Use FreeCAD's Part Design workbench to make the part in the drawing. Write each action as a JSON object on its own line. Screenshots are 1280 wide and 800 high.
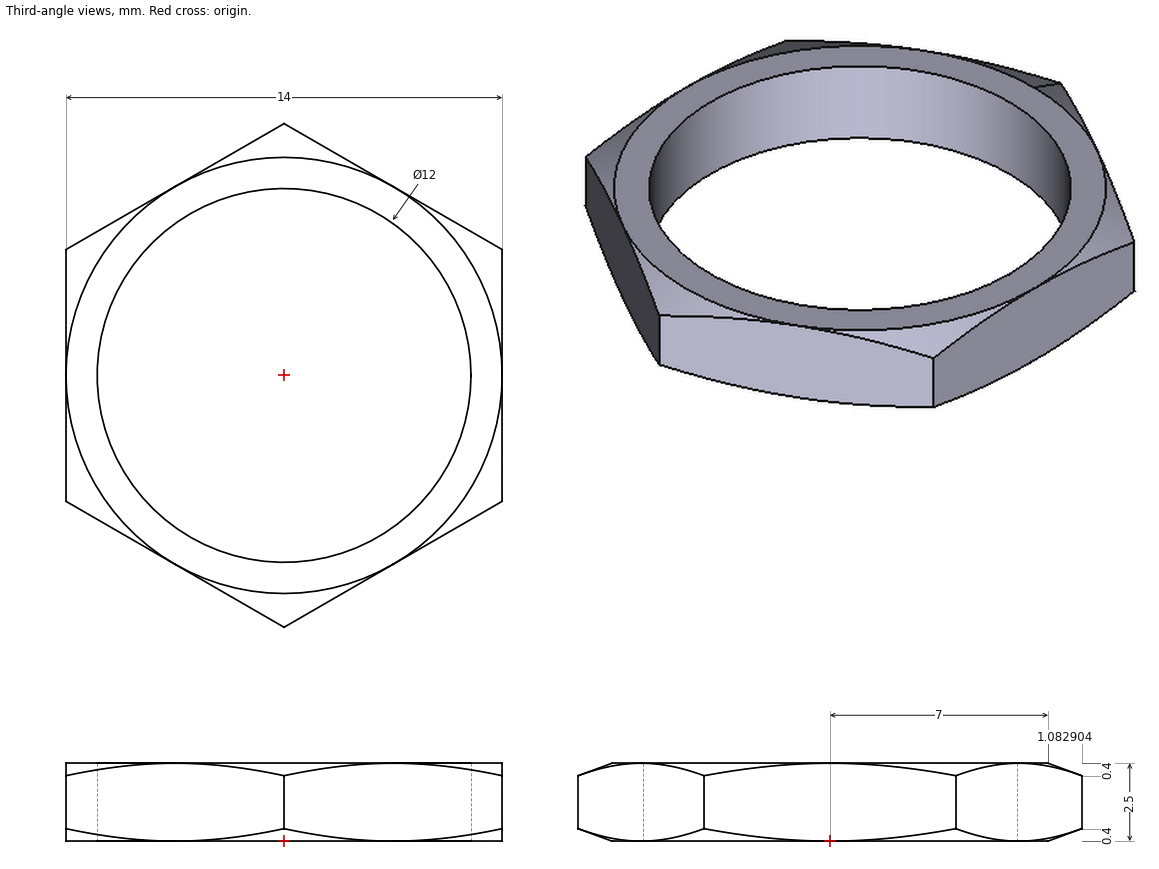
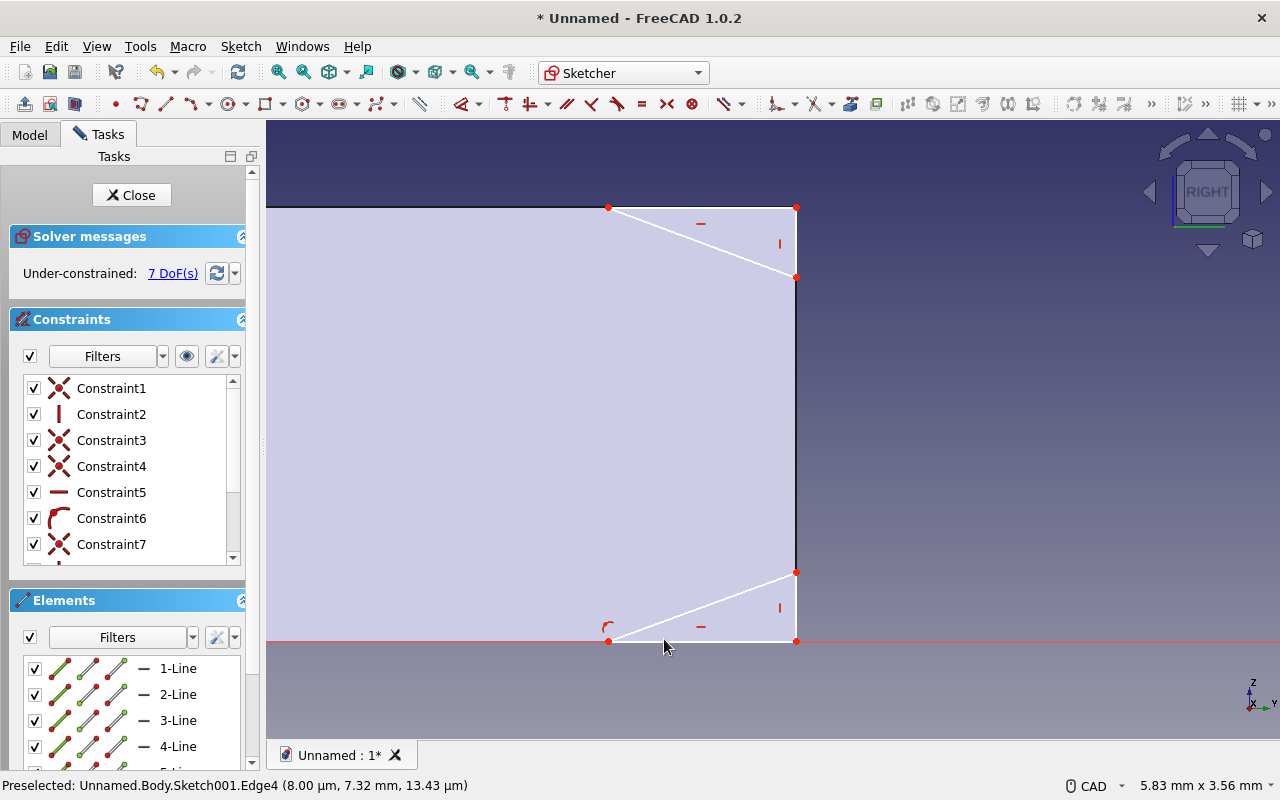
{"action": "key", "text": "d"}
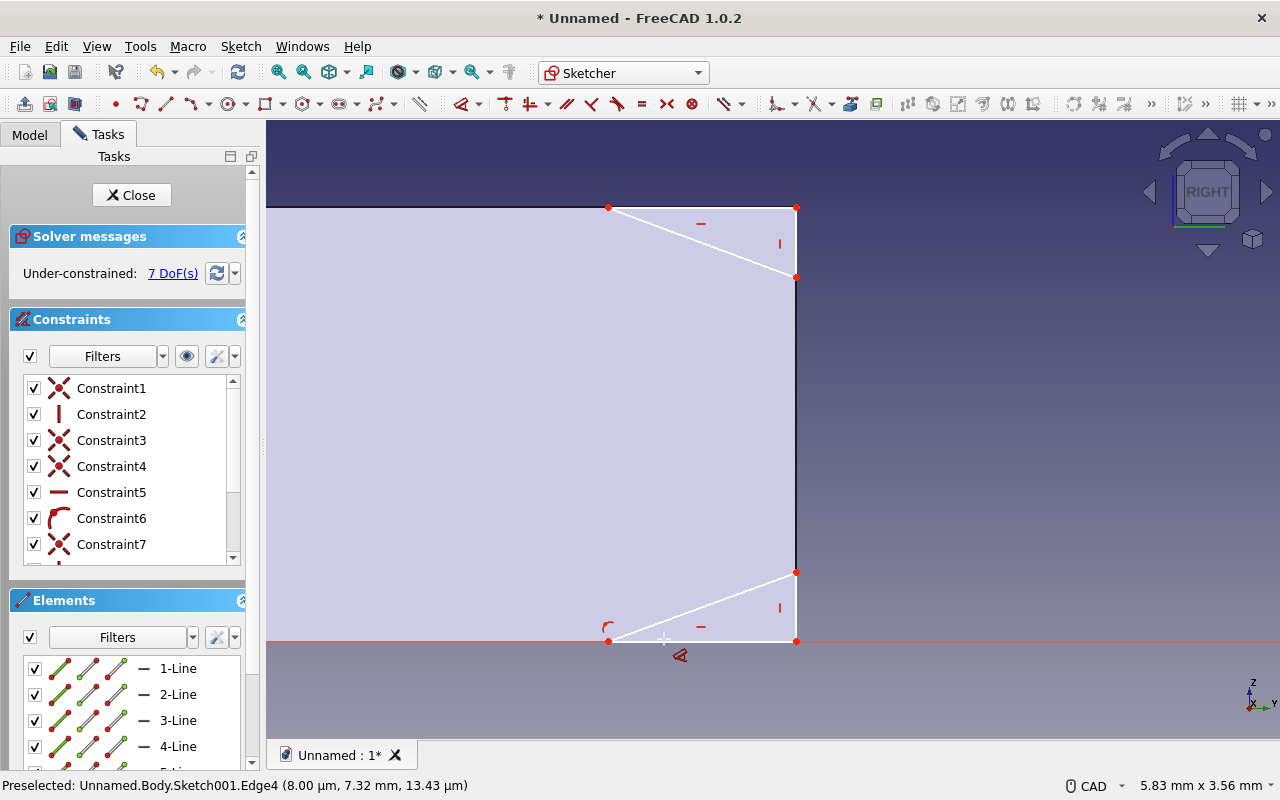
{"action": "left_click", "coordinate": [608, 208]}
{"action": "left_click", "coordinate": [451, 676]}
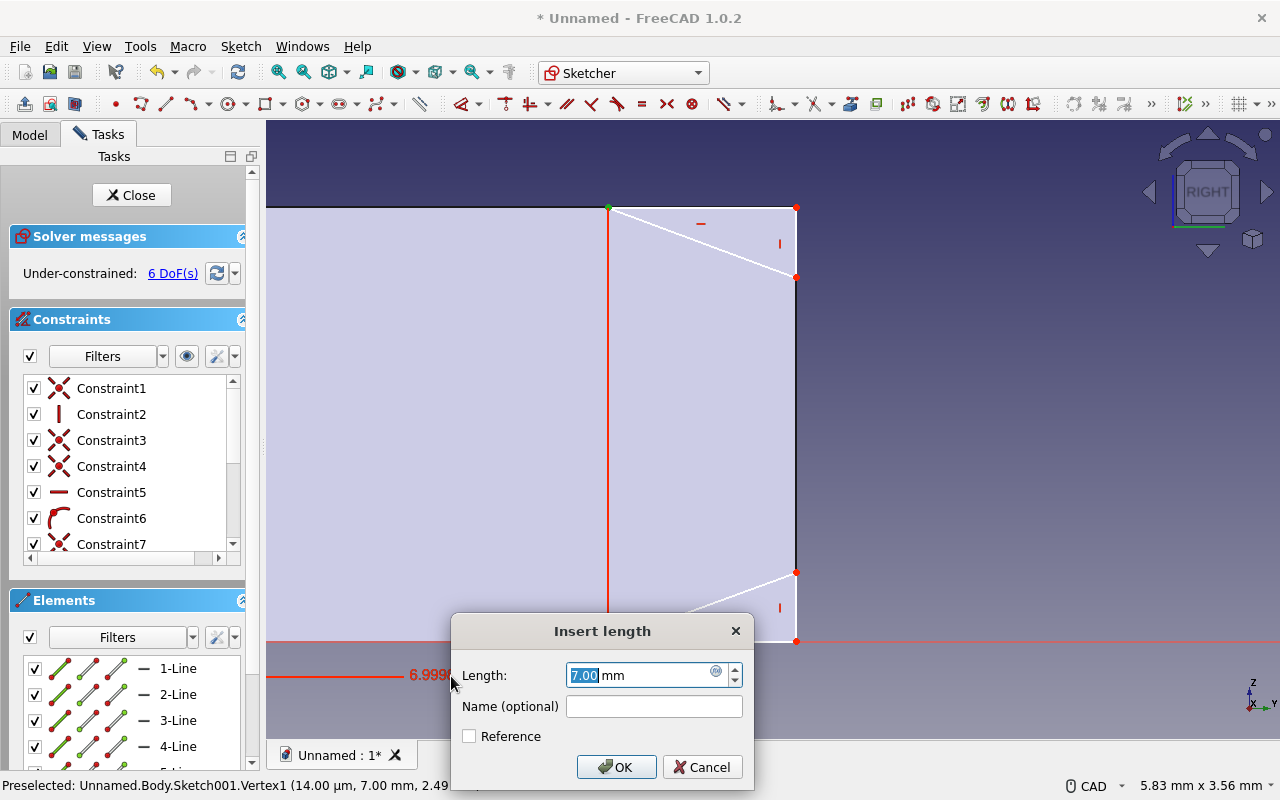
{"action": "type", "text": "7"}
{"action": "key", "text": "Return"}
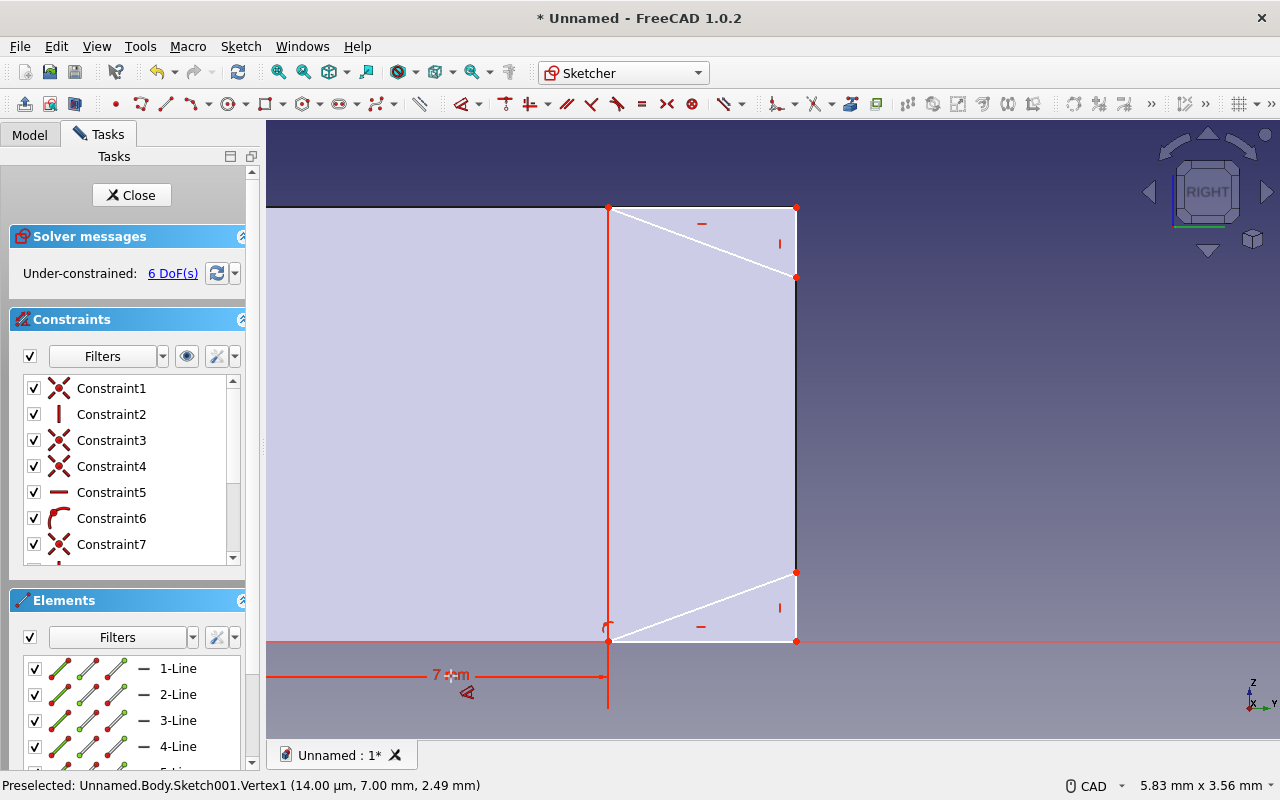
{"action": "left_click", "coordinate": [608, 642]}
{"action": "left_click", "coordinate": [379, 676]}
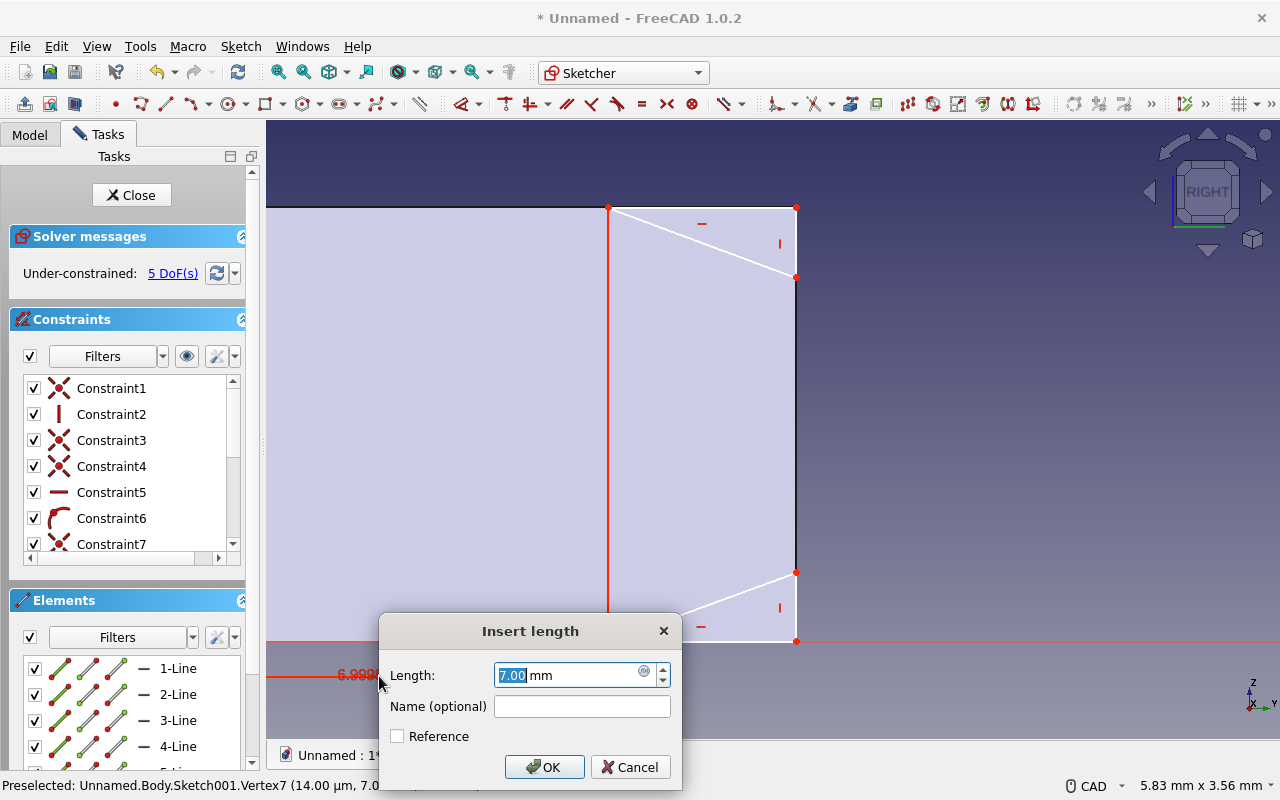
{"action": "type", "text": "7"}
{"action": "key", "text": "Return"}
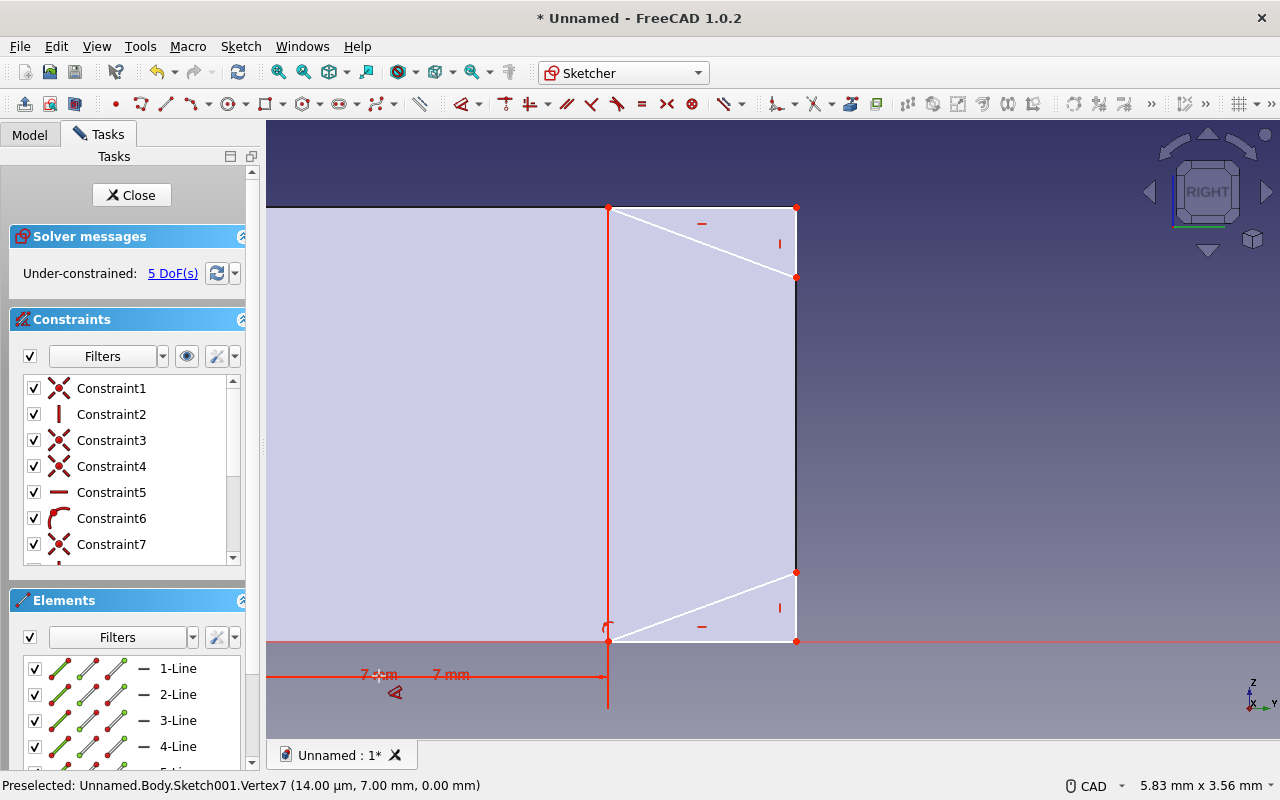
{"action": "left_click", "coordinate": [796, 257]}
{"action": "left_click", "coordinate": [830, 243]}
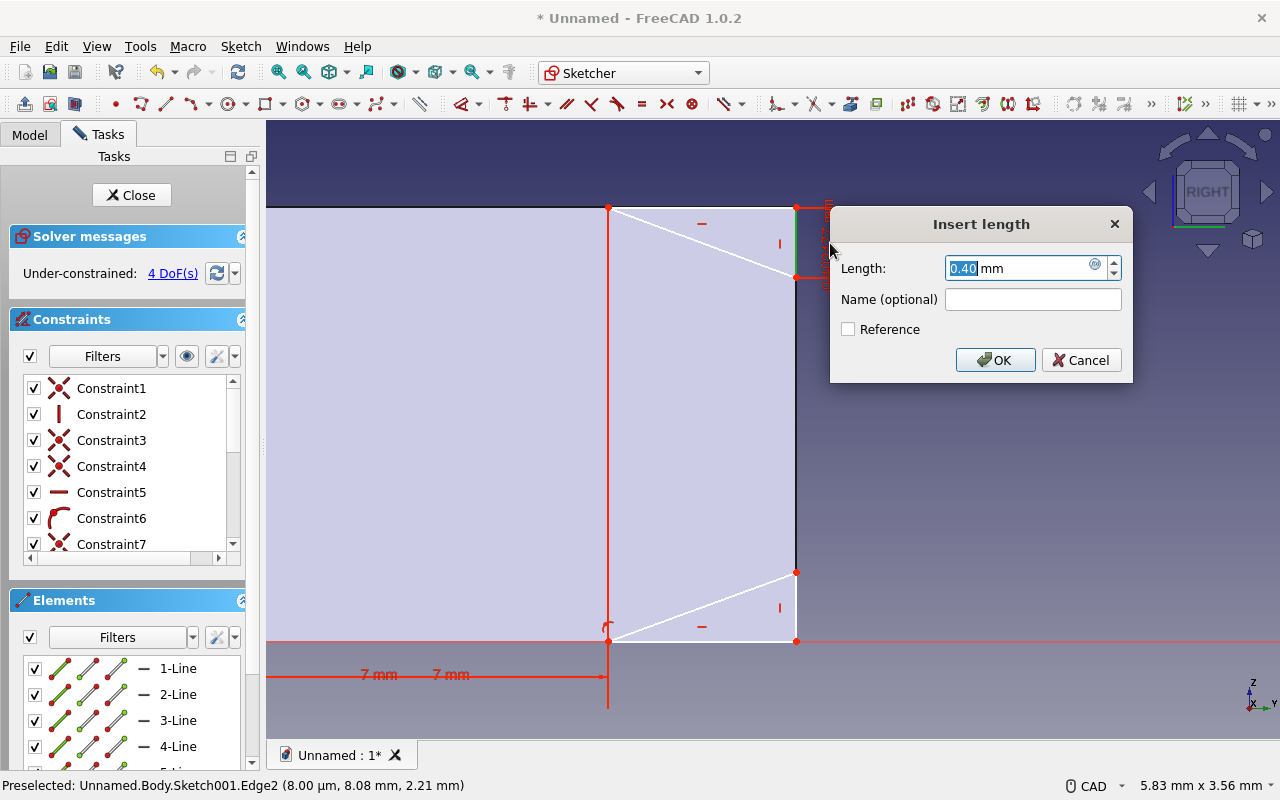
{"action": "type", "text": "0.4"}
{"action": "key", "text": "Return"}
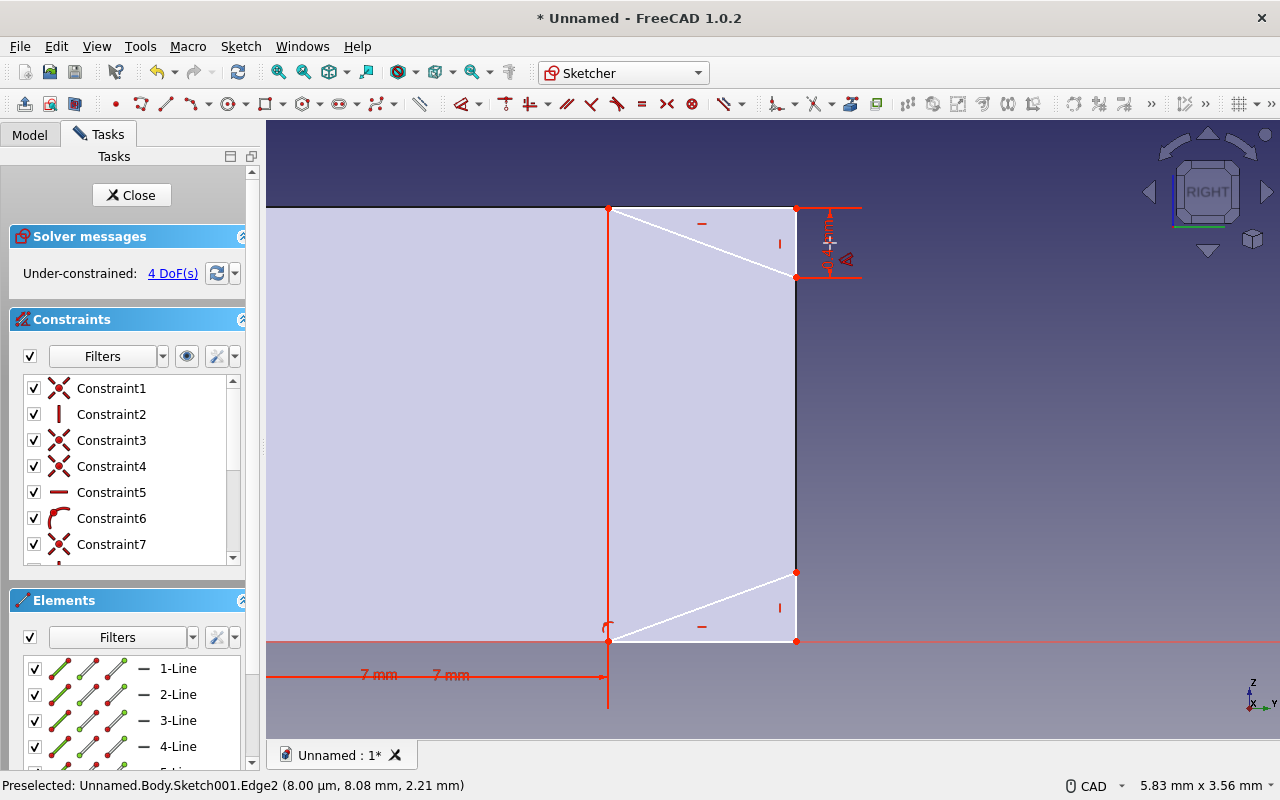
{"action": "left_click", "coordinate": [796, 621]}
{"action": "left_click", "coordinate": [830, 607]}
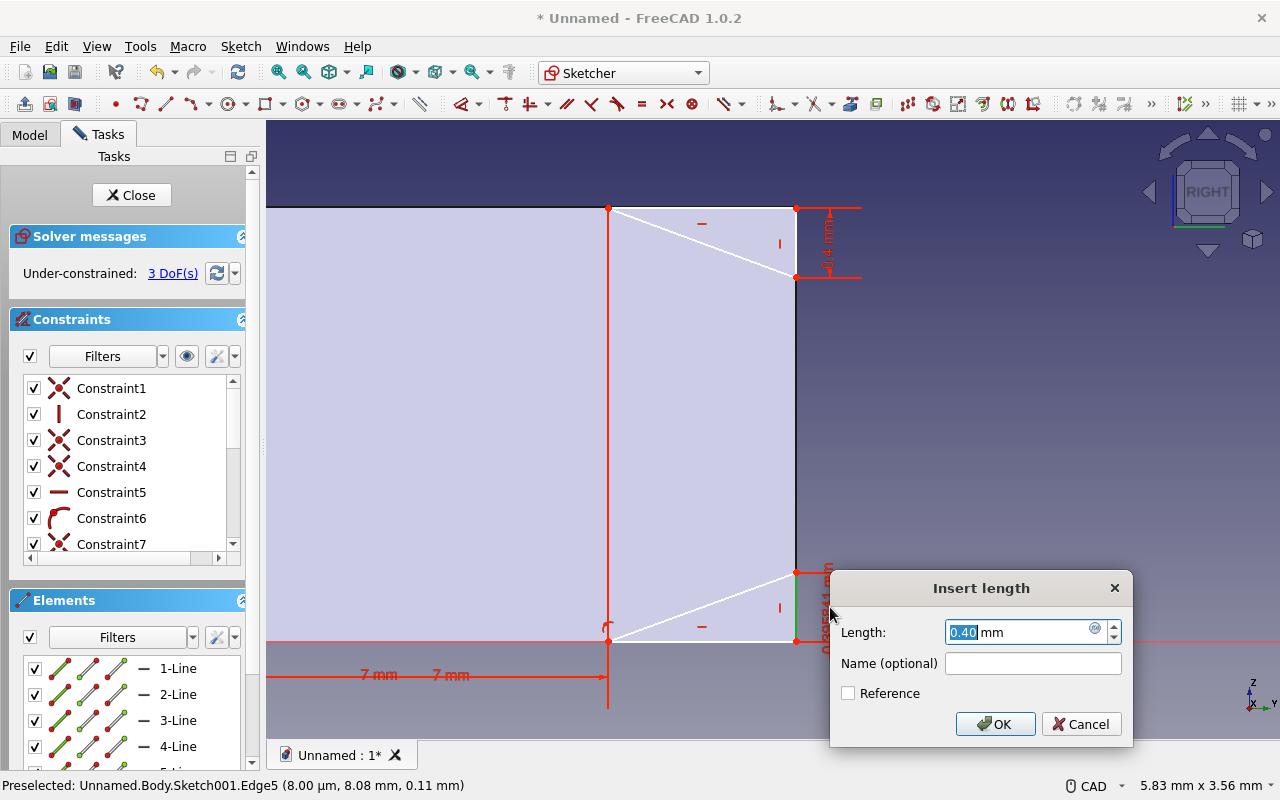
{"action": "type", "text": "0.4"}
{"action": "key", "text": "Return"}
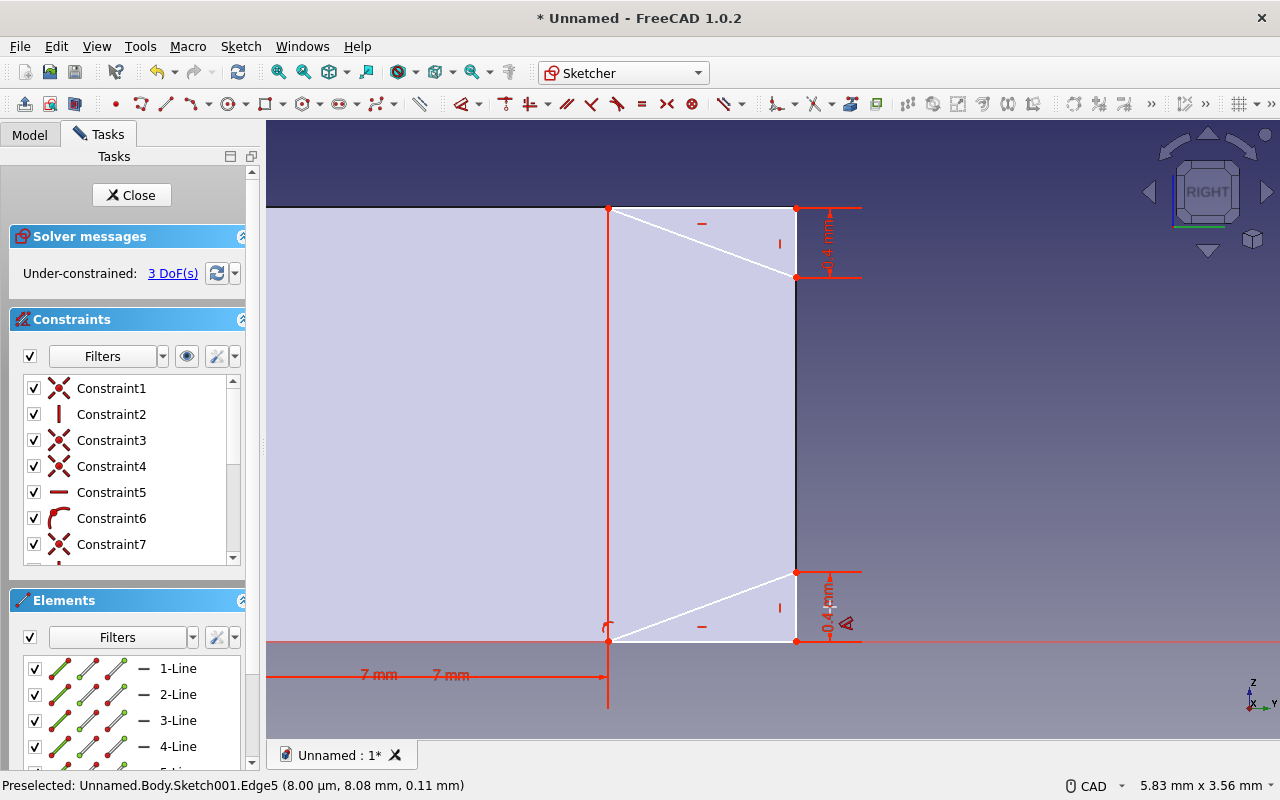
{"action": "left_click", "coordinate": [608, 208]}
{"action": "left_click", "coordinate": [642, 425]}